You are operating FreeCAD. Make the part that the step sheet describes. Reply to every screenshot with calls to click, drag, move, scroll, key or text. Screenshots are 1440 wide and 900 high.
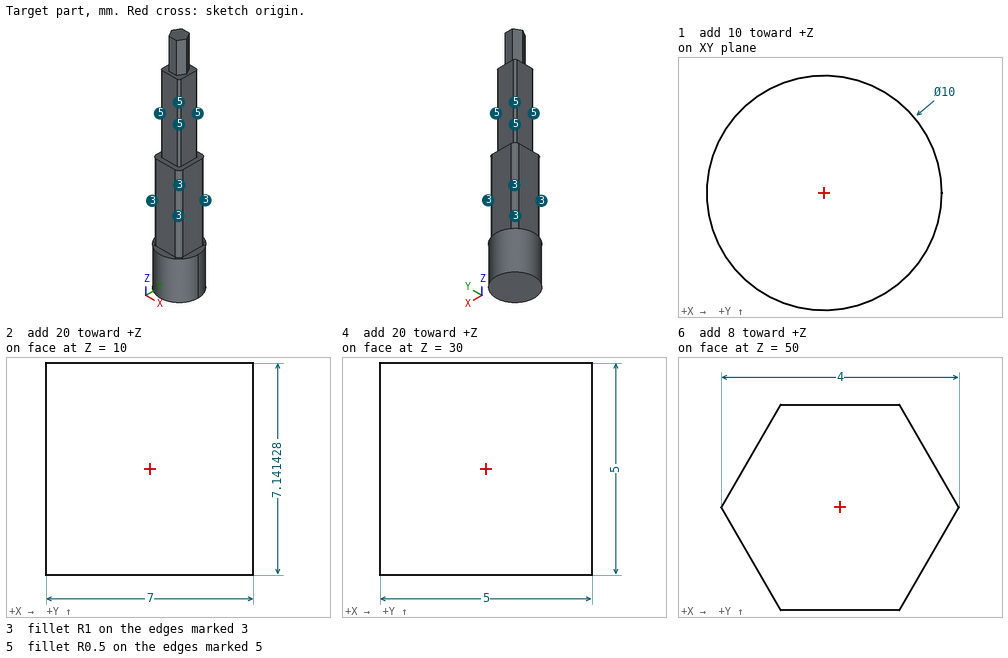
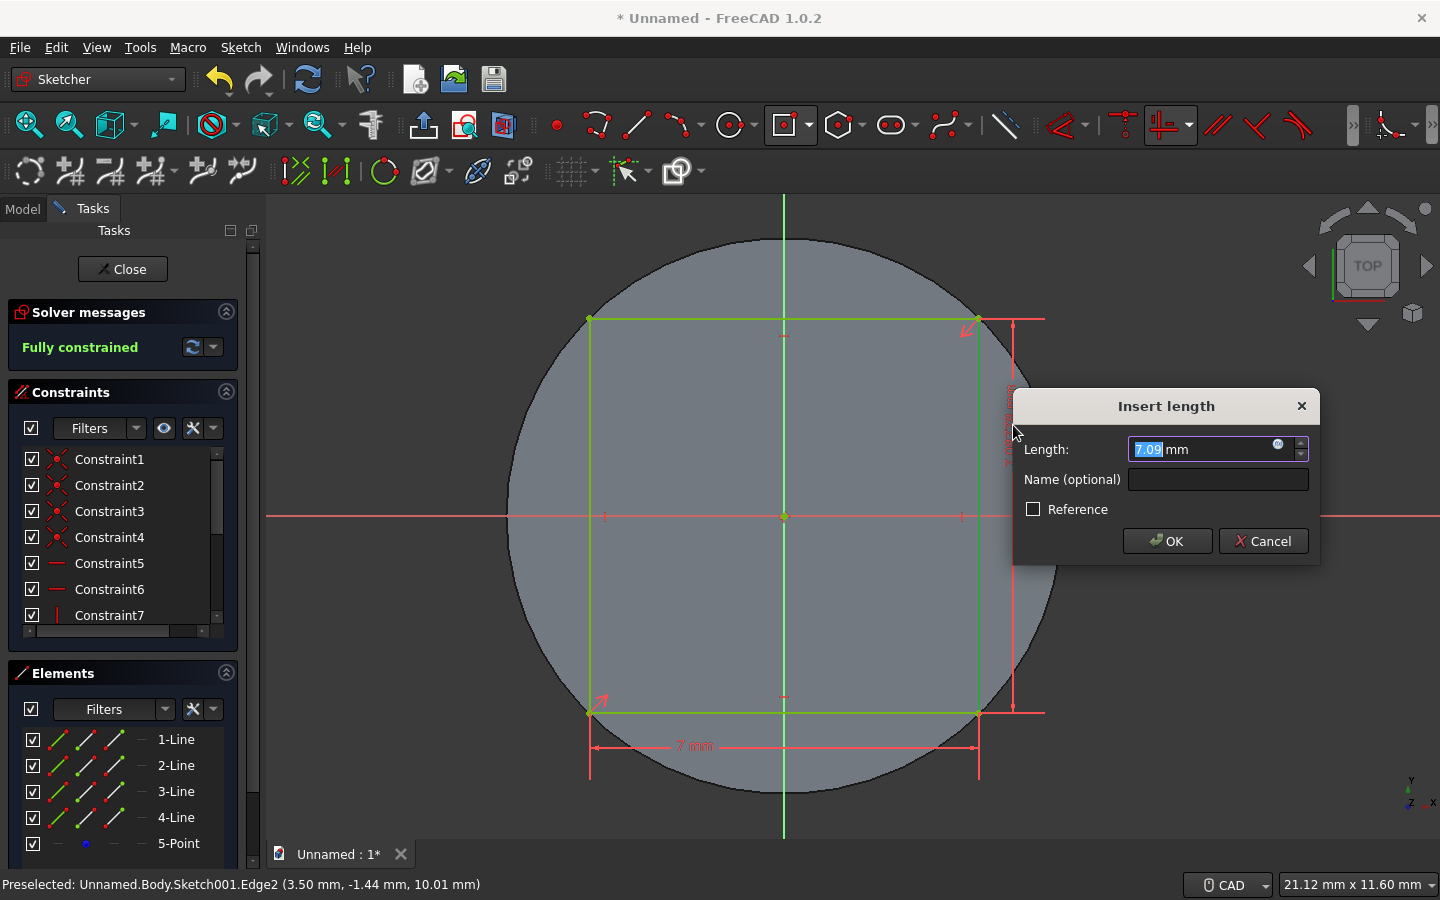
text(7.141428)
key(Return)
key(Escape)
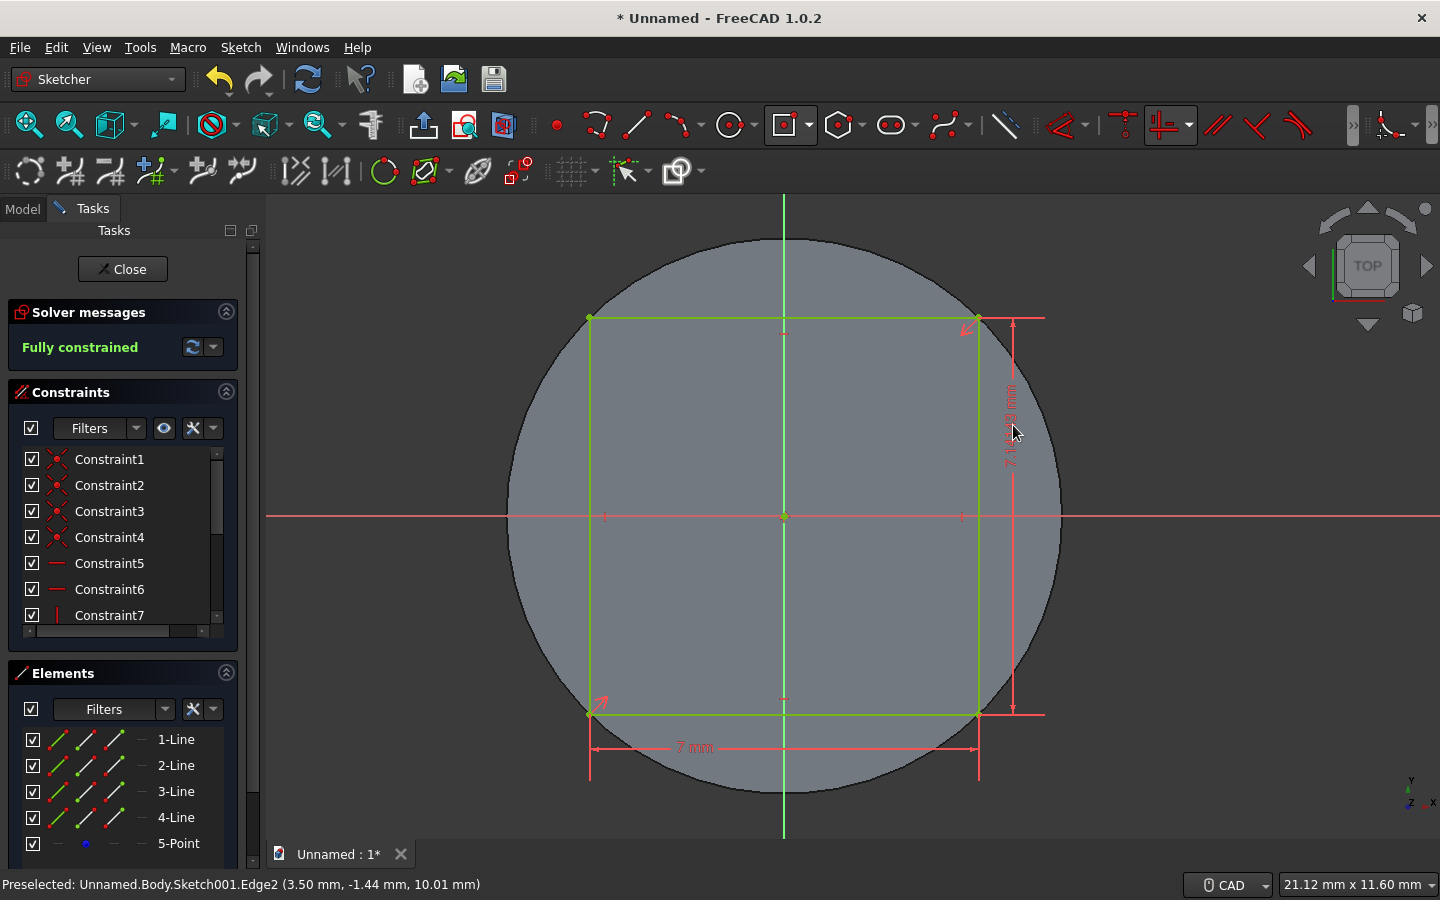
click(123, 269)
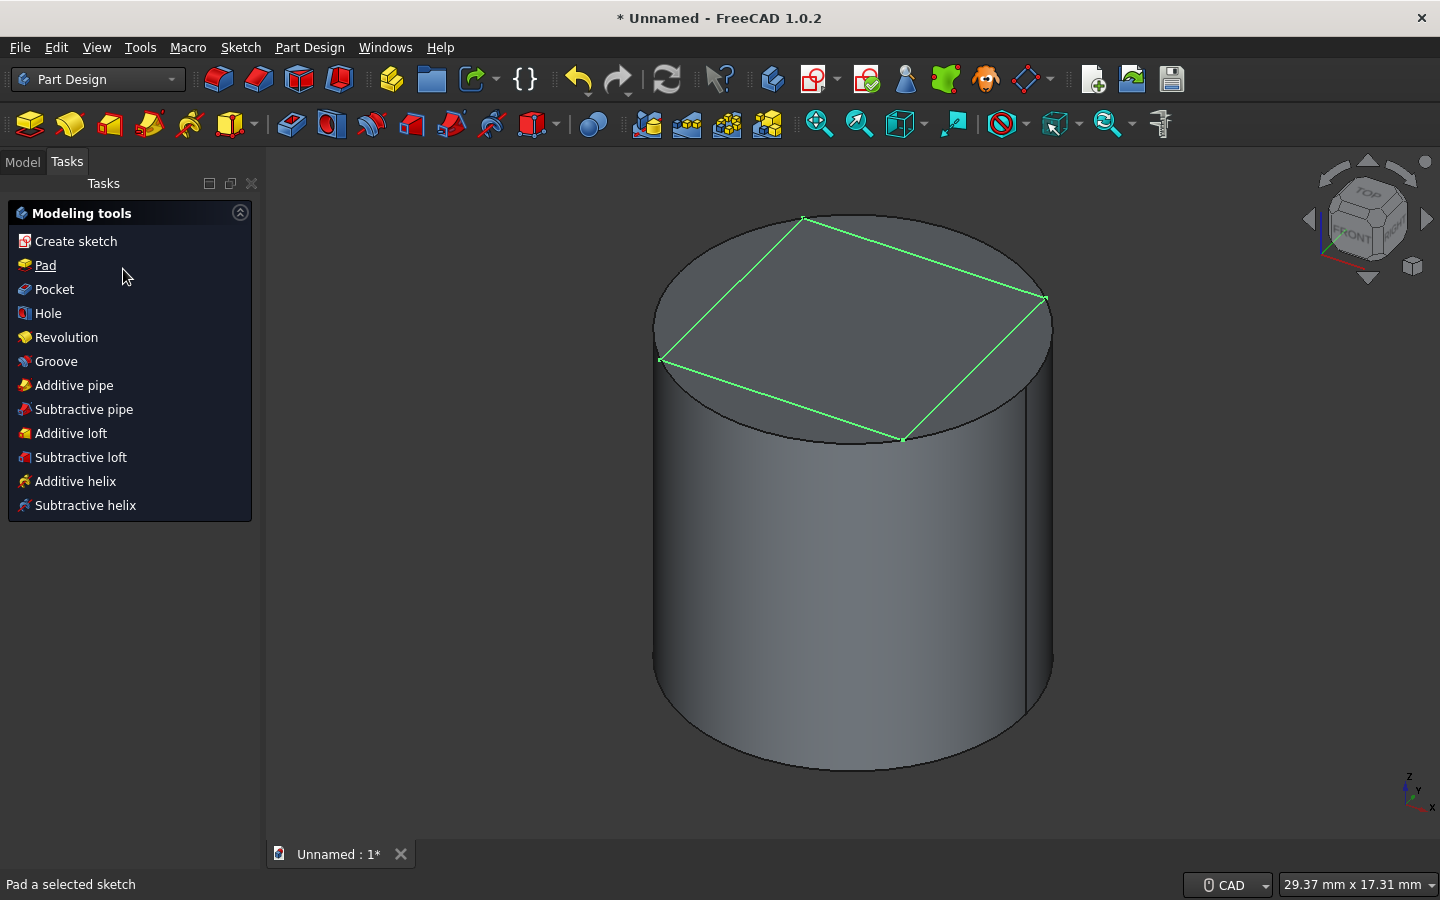
click(30, 124)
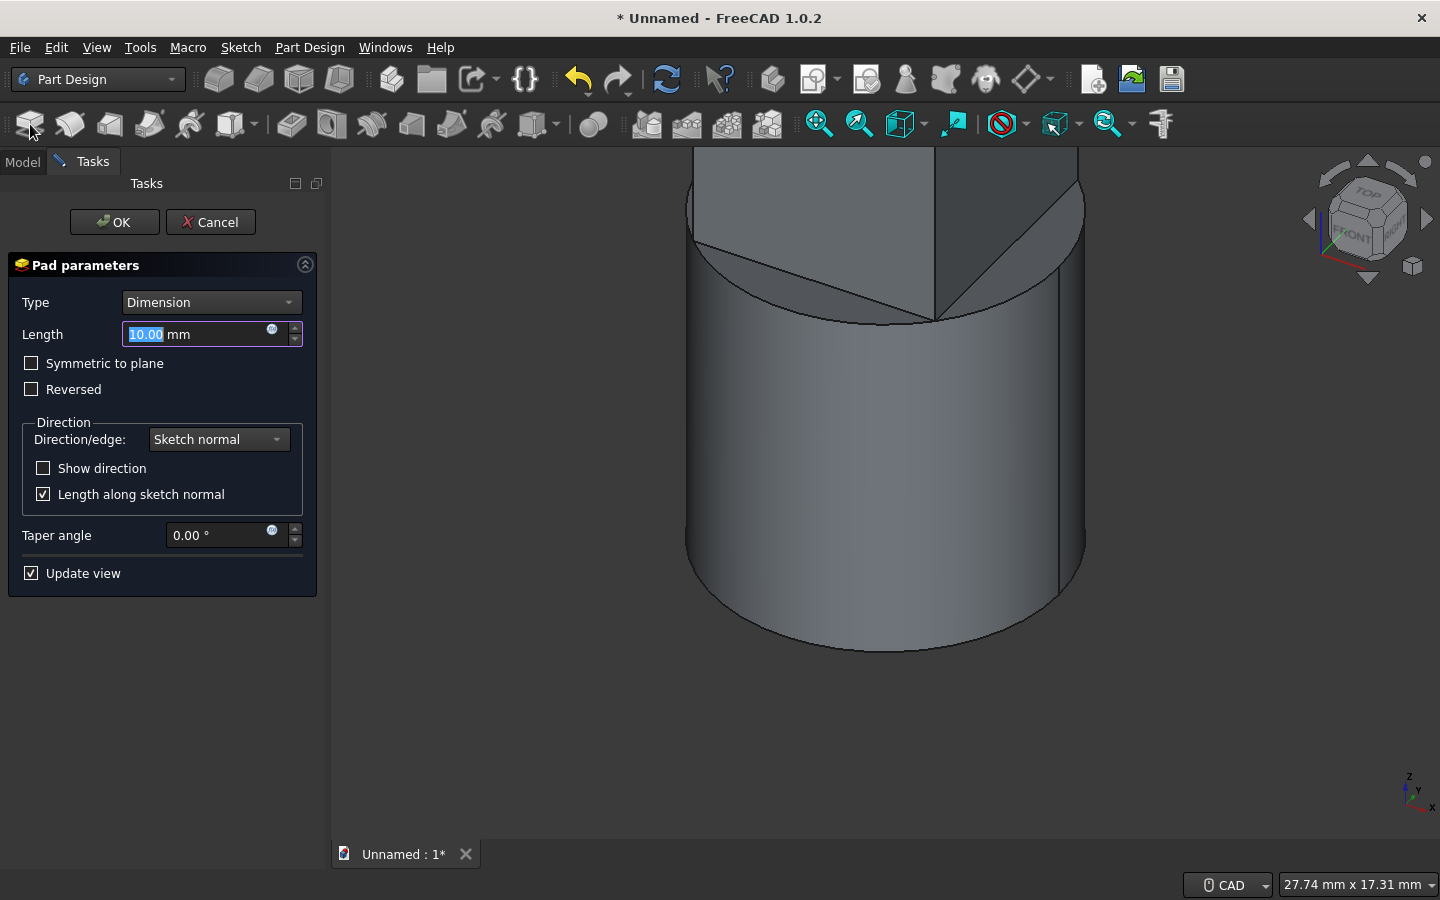
text(20)
key(Tab)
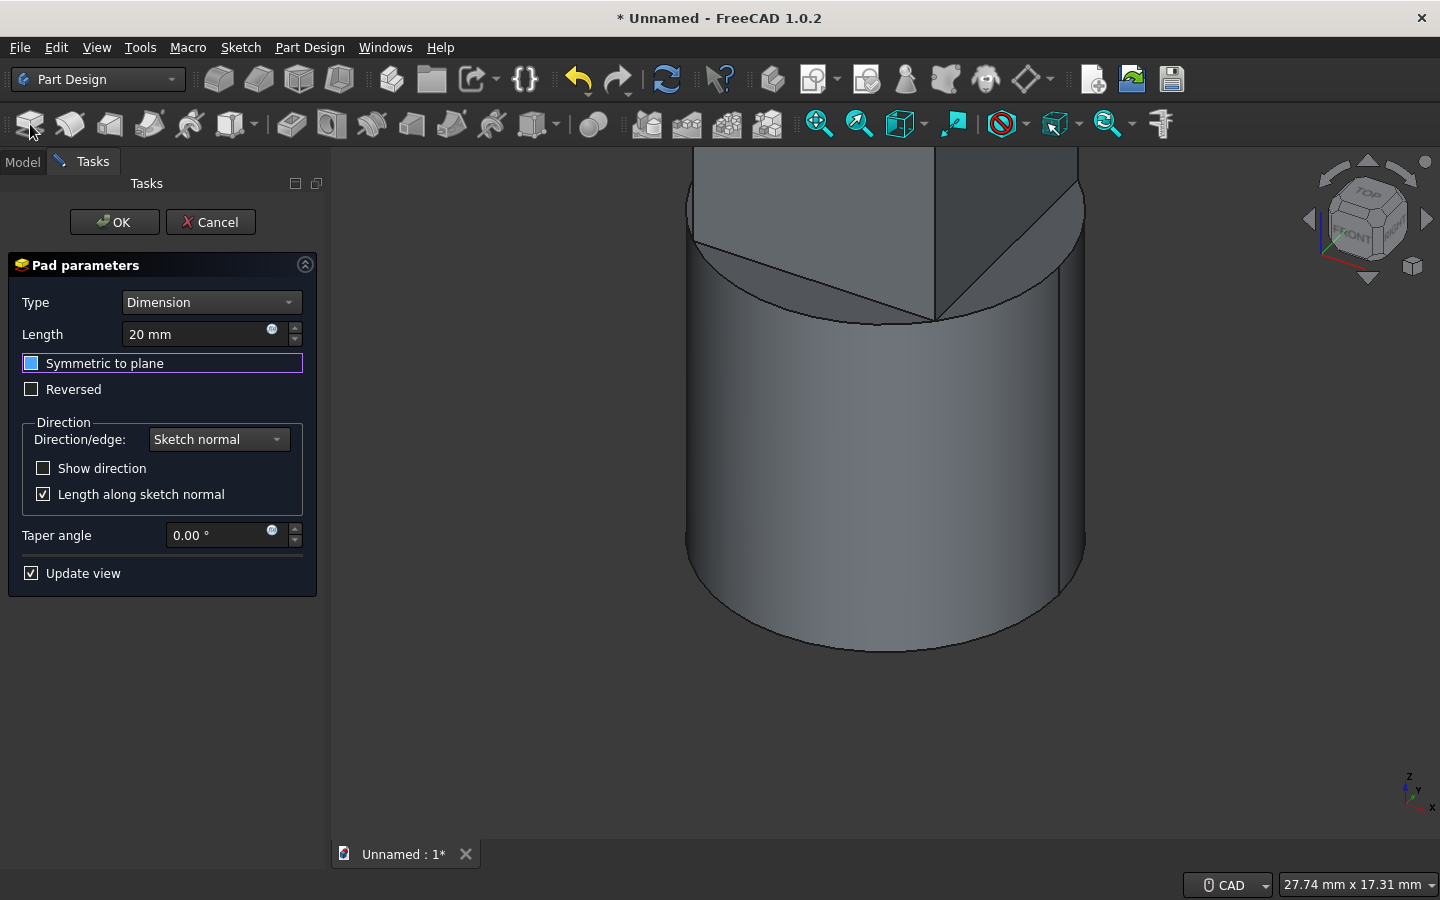
click(115, 222)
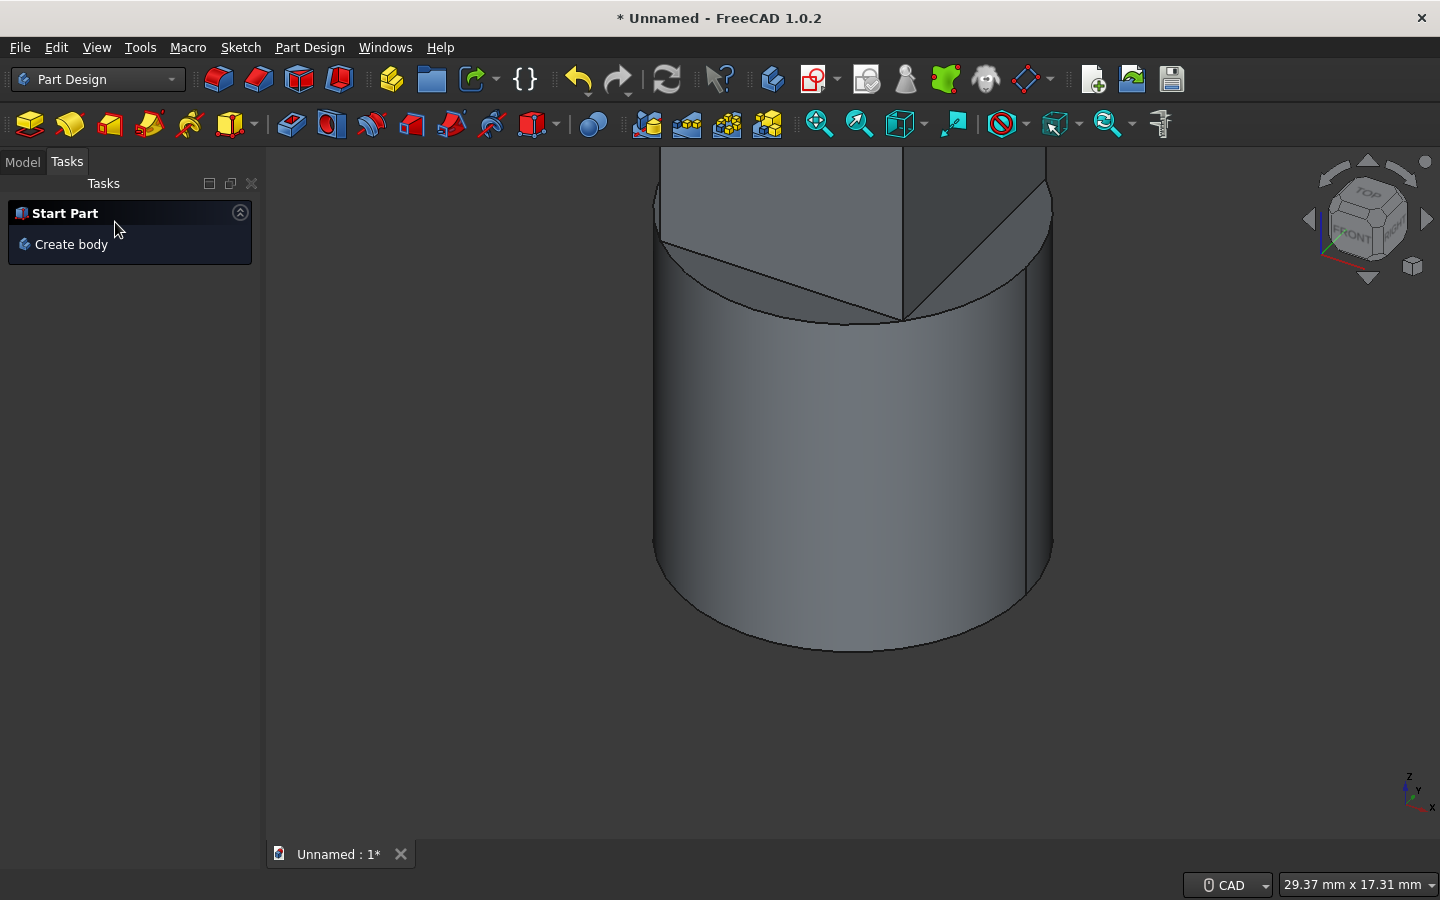
click(820, 124)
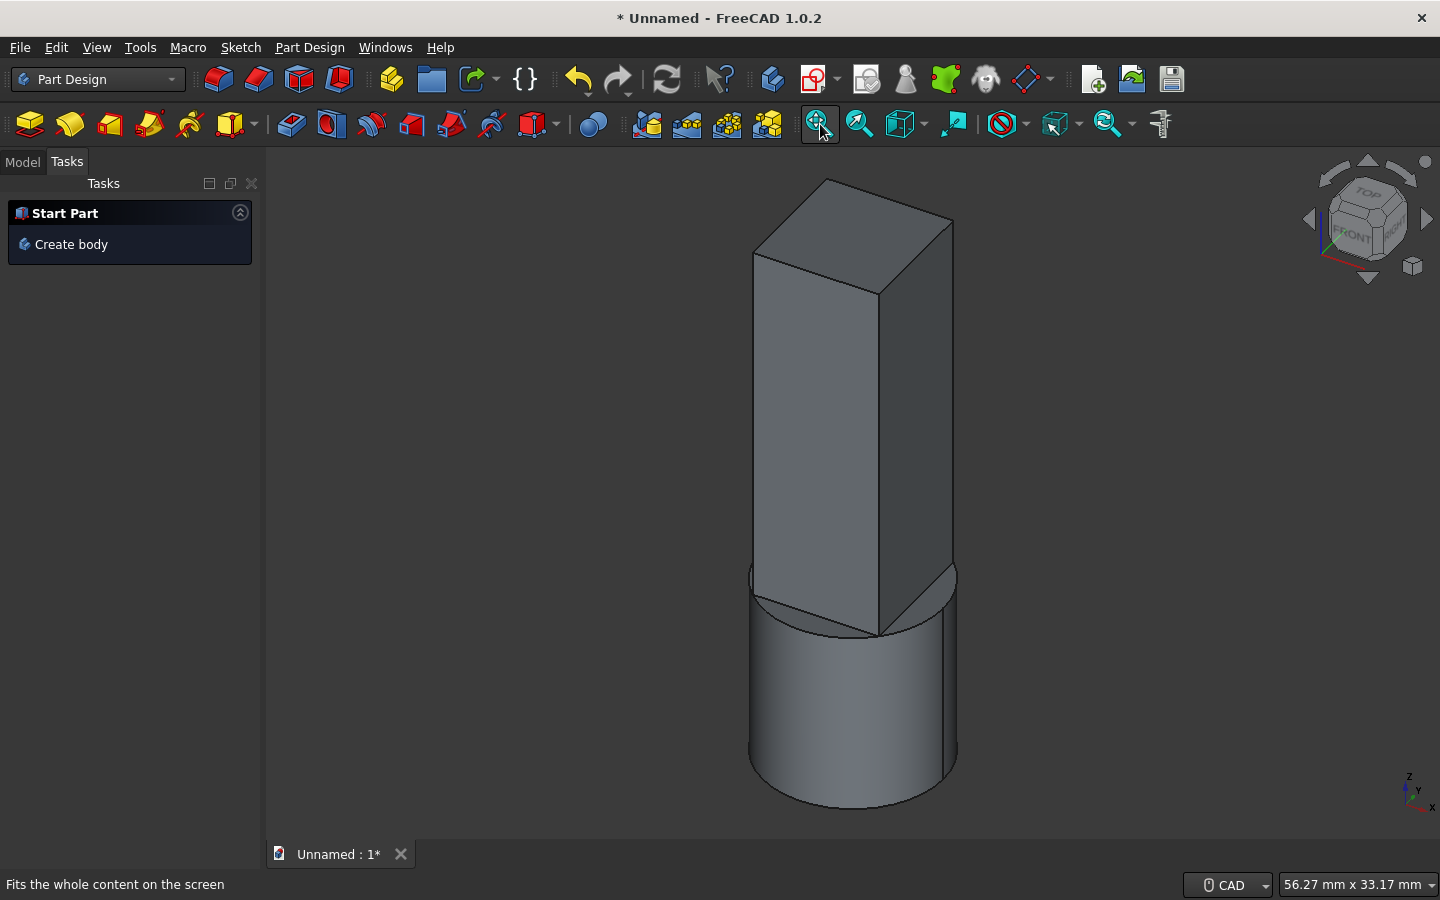
click(879, 464)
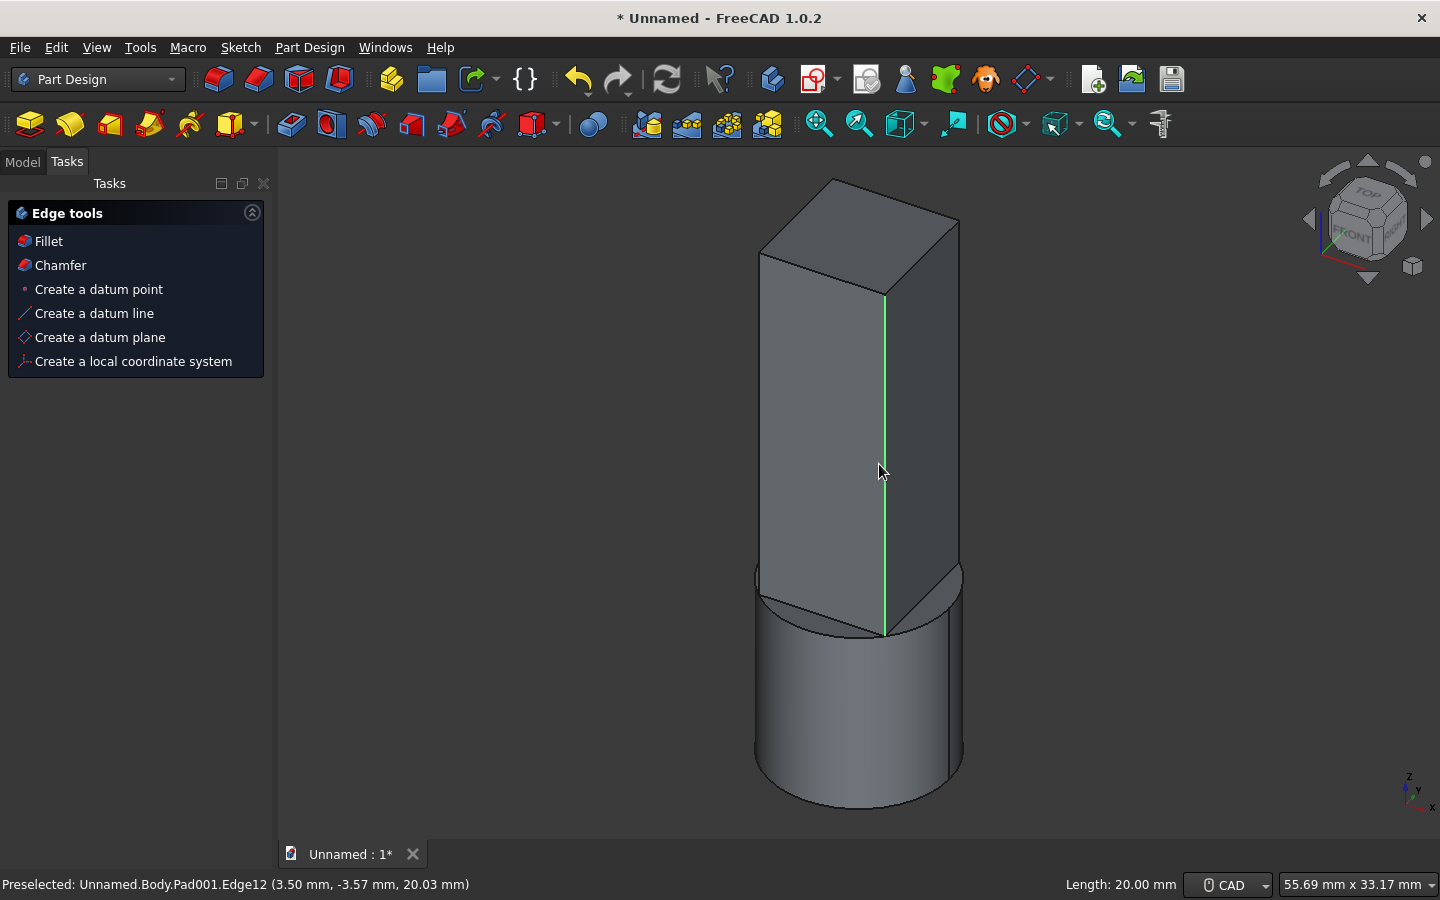
key(0)